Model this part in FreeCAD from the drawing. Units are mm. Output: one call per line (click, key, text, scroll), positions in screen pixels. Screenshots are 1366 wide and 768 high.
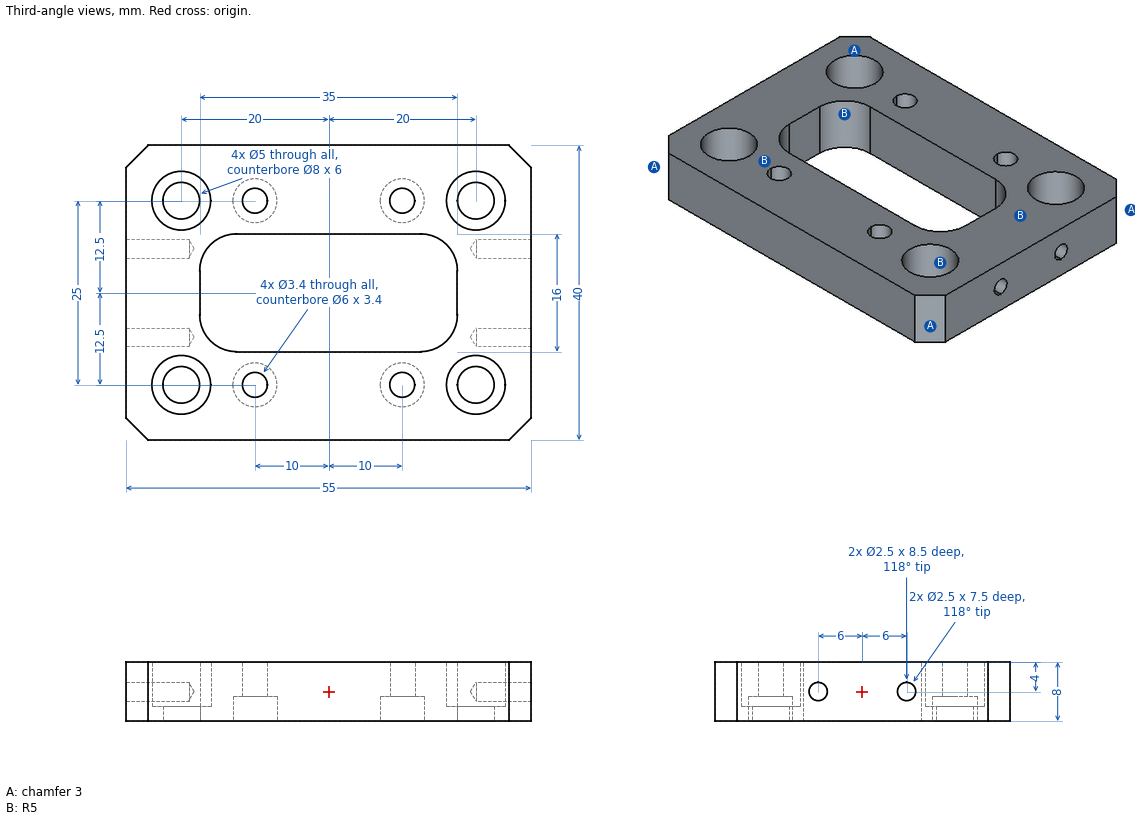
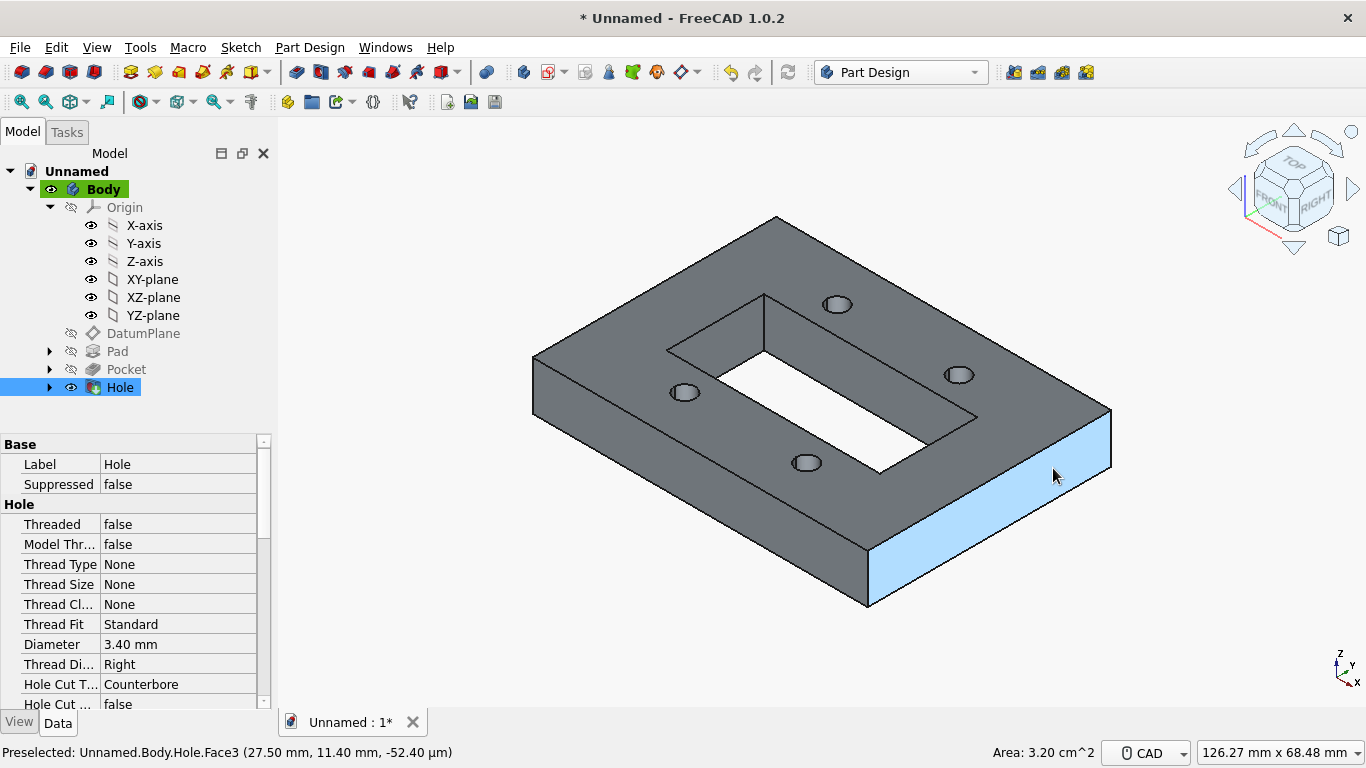
click(548, 72)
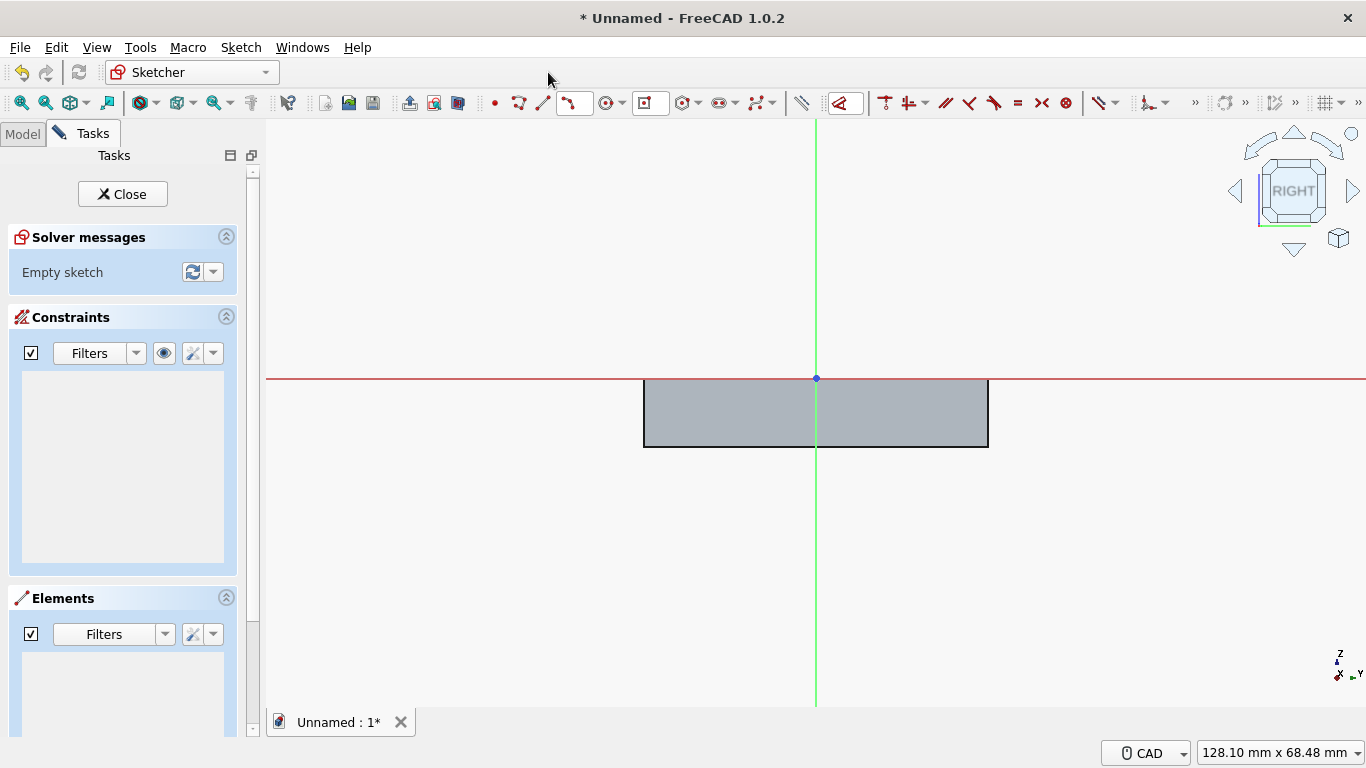
scroll(833, 398, up, 8)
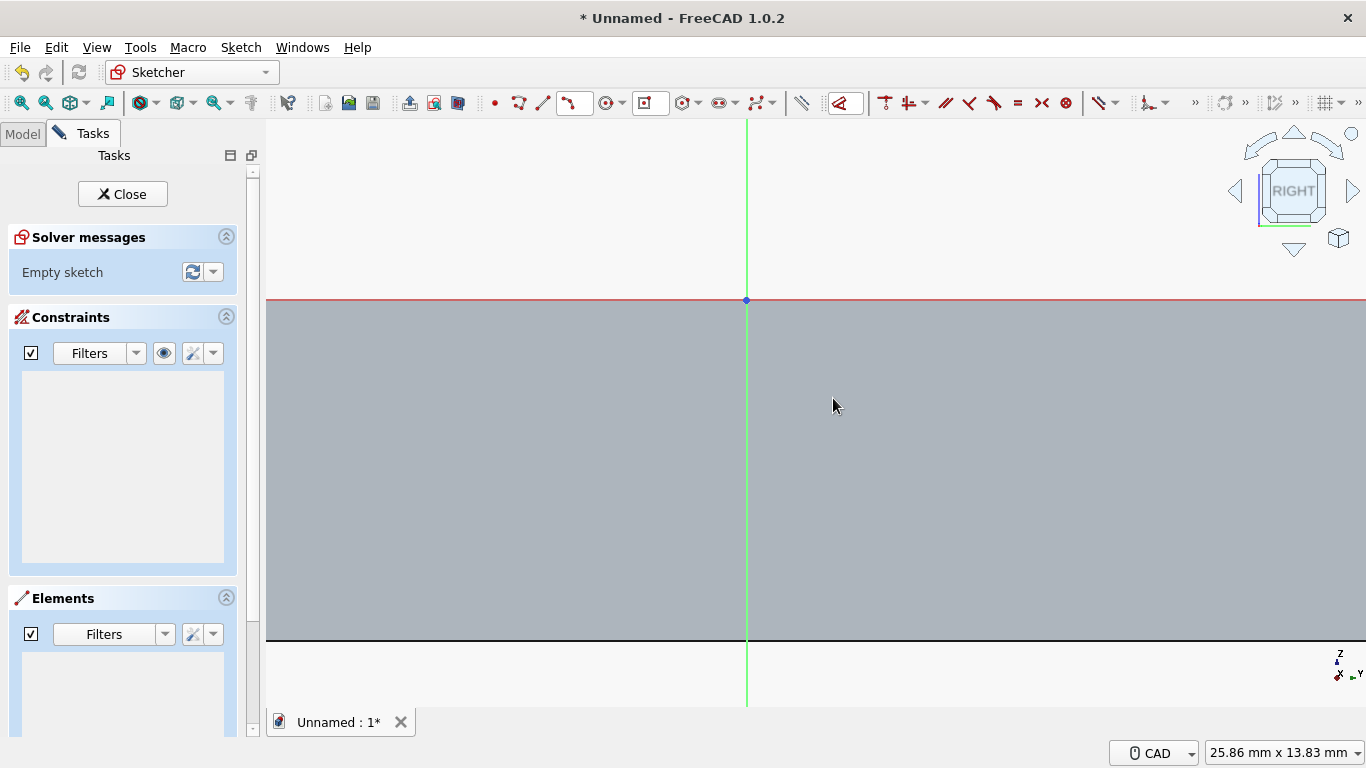
click(606, 104)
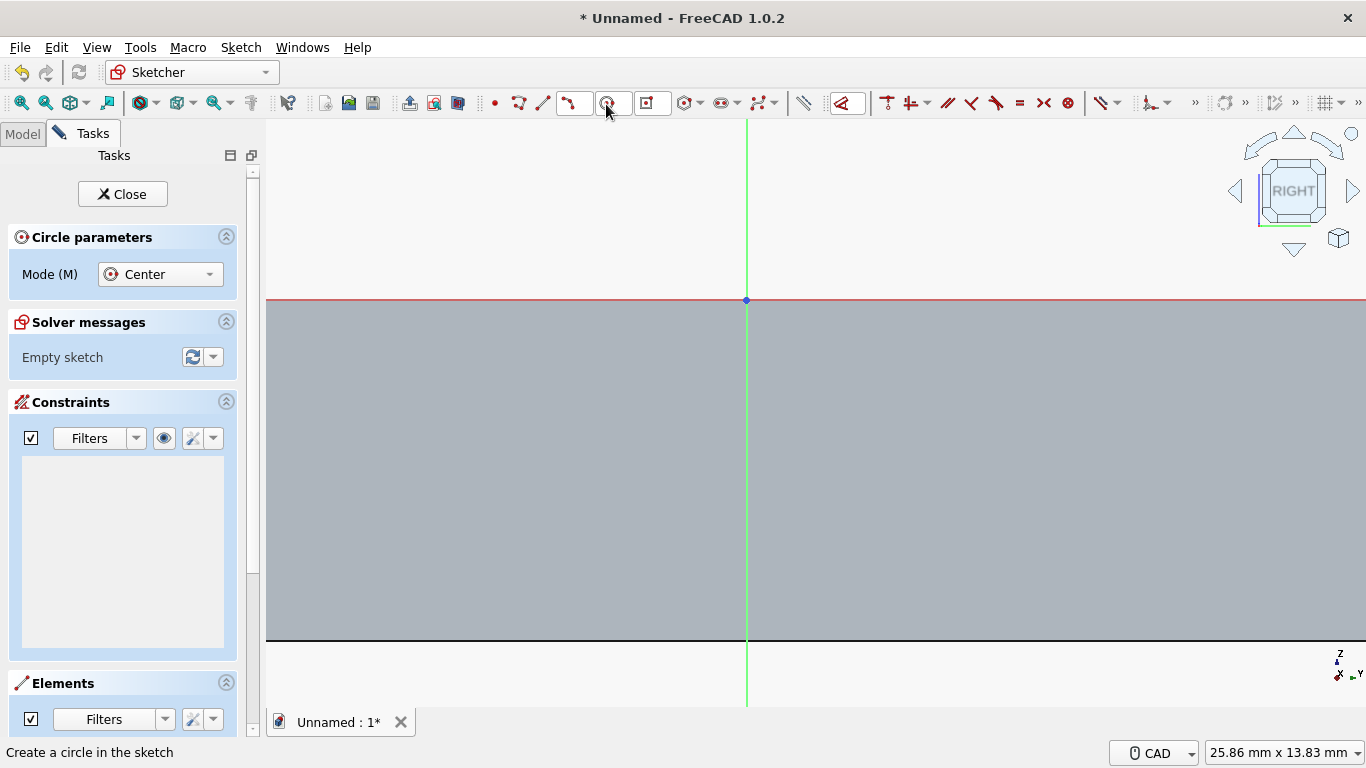
click(1002, 470)
move(1040, 433)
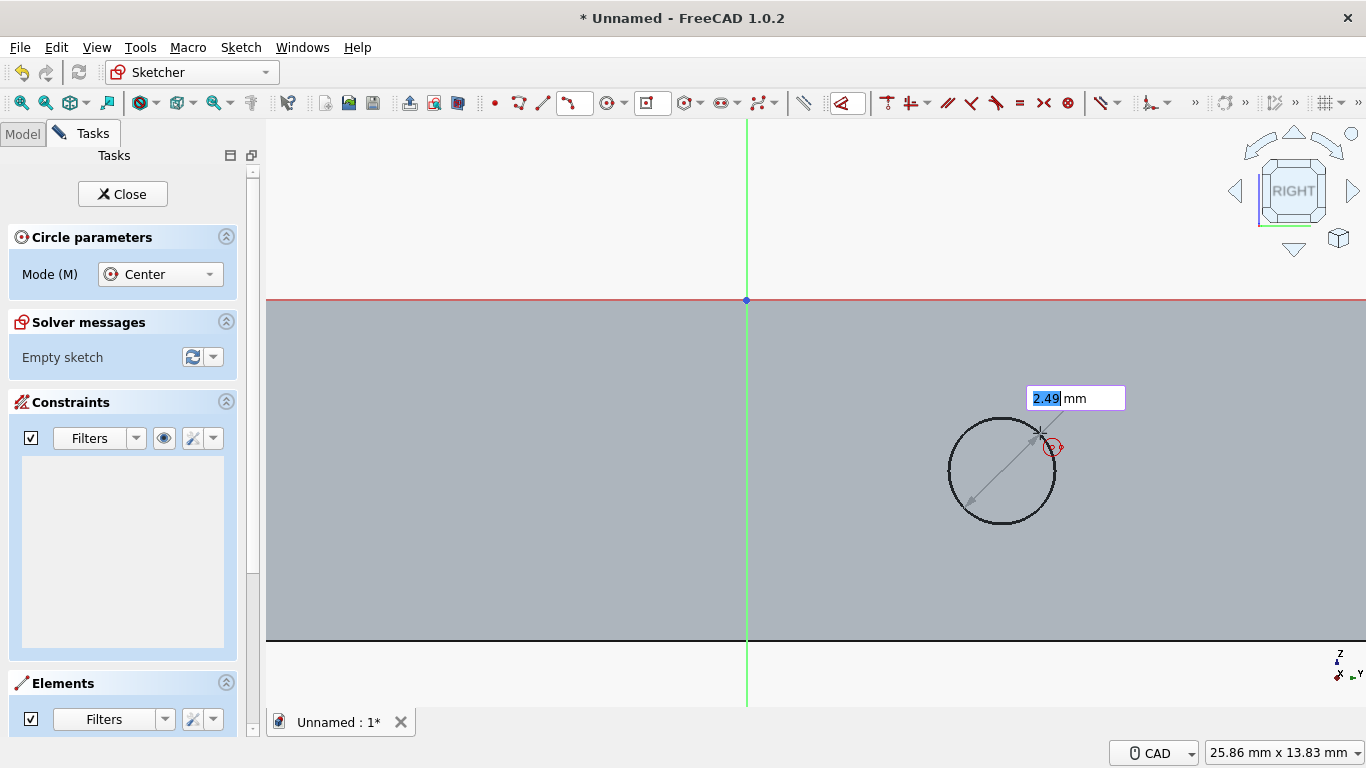
text(2.5)
key(Return)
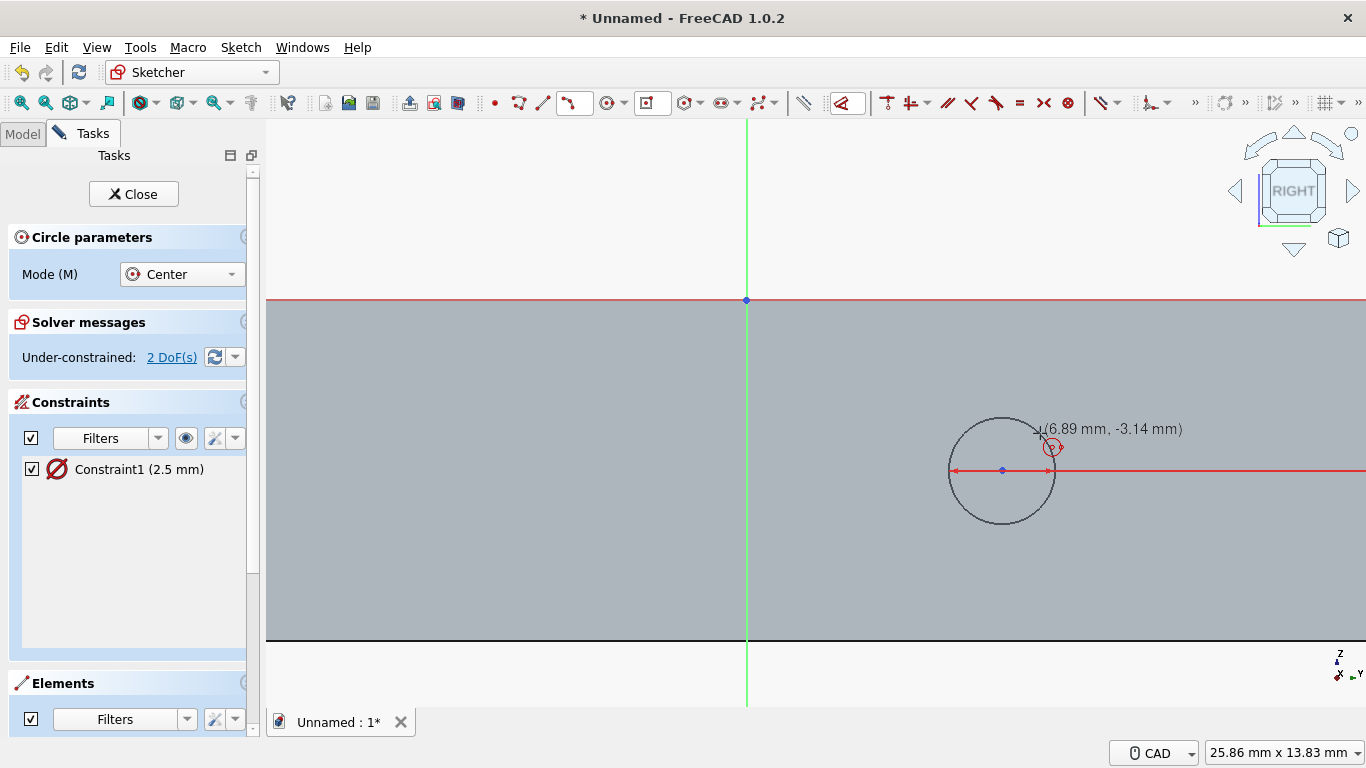
click(492, 470)
move(529, 433)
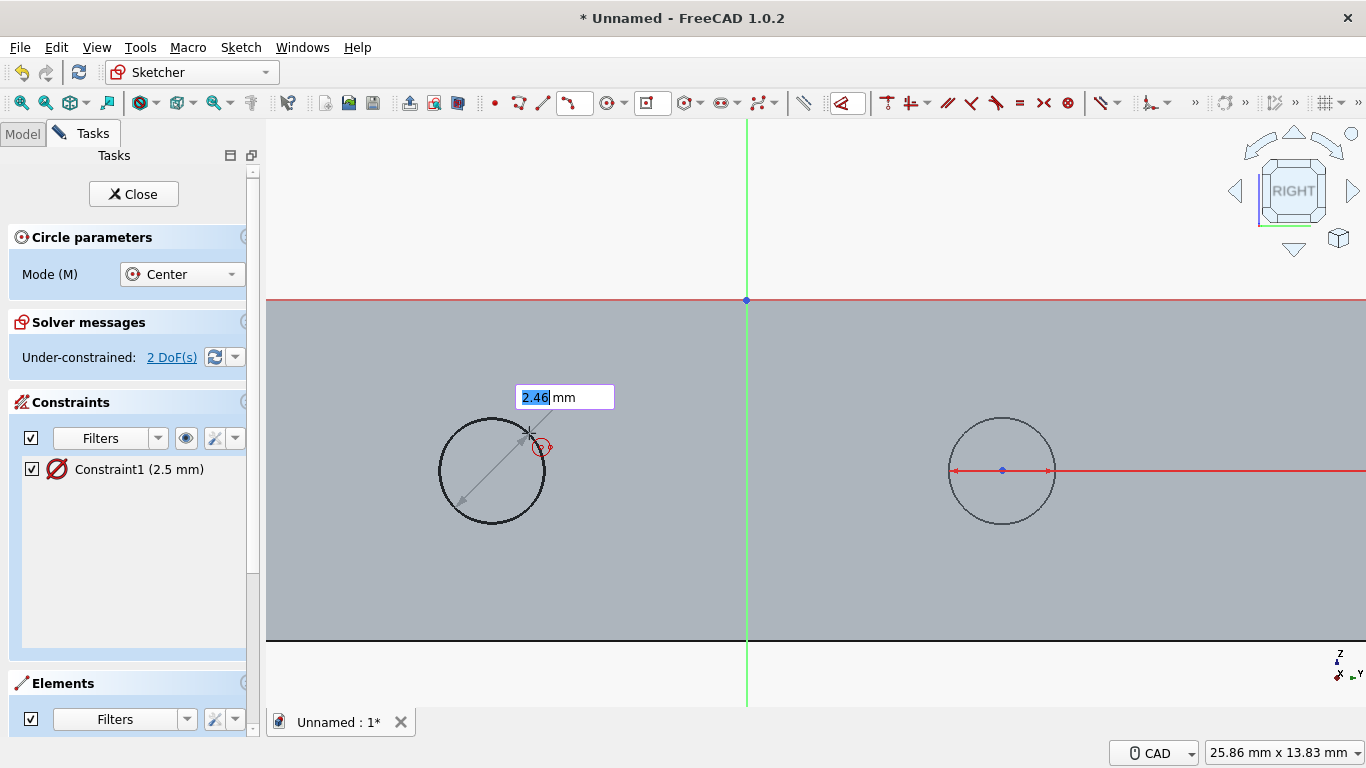
text(2.5)
key(Return)
key(Escape)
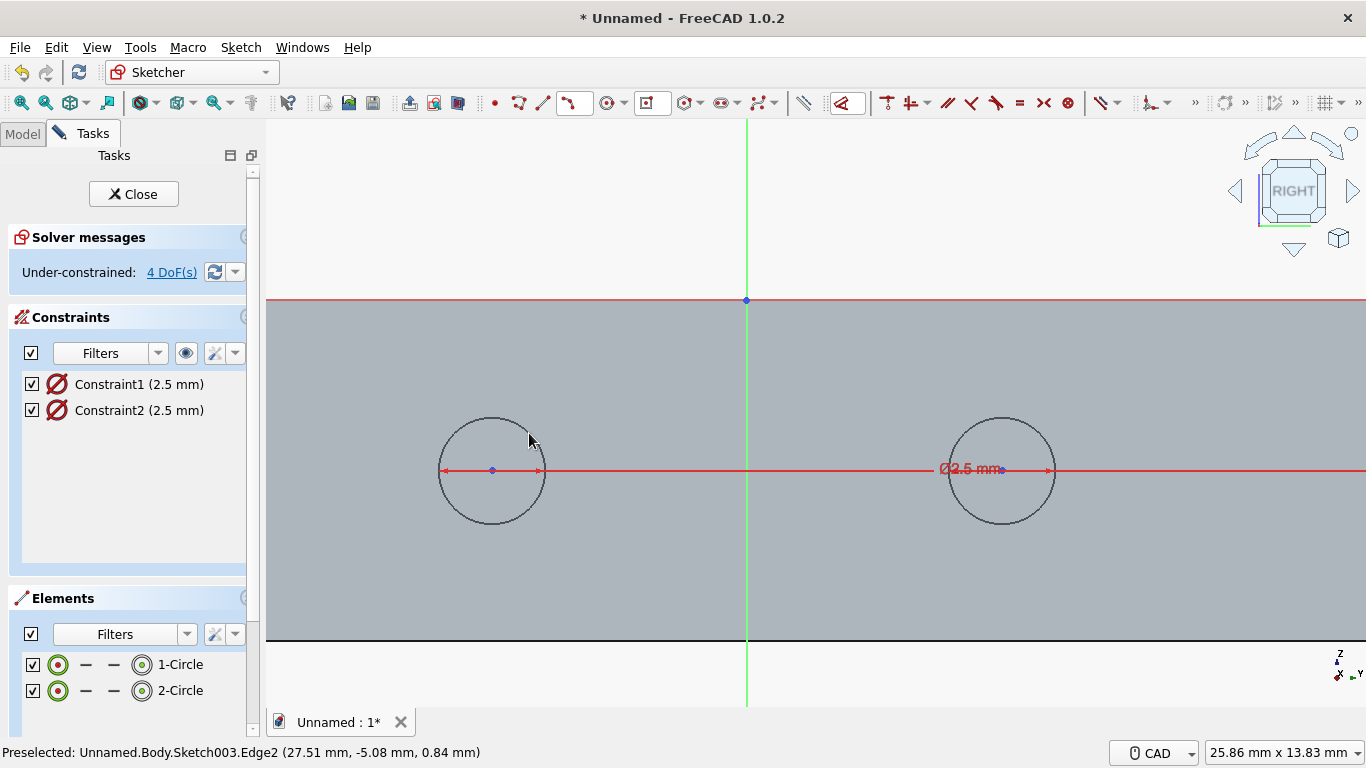
click(1002, 471)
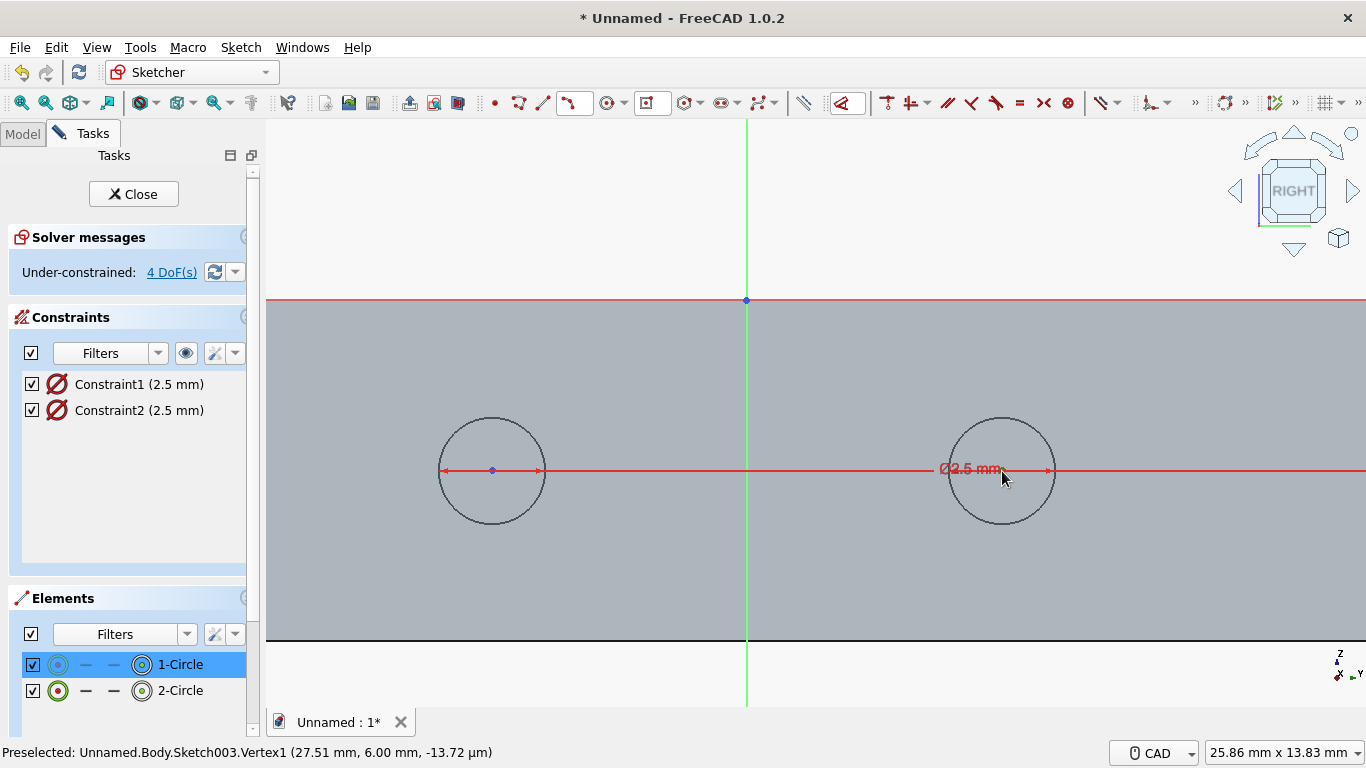
click(492, 471)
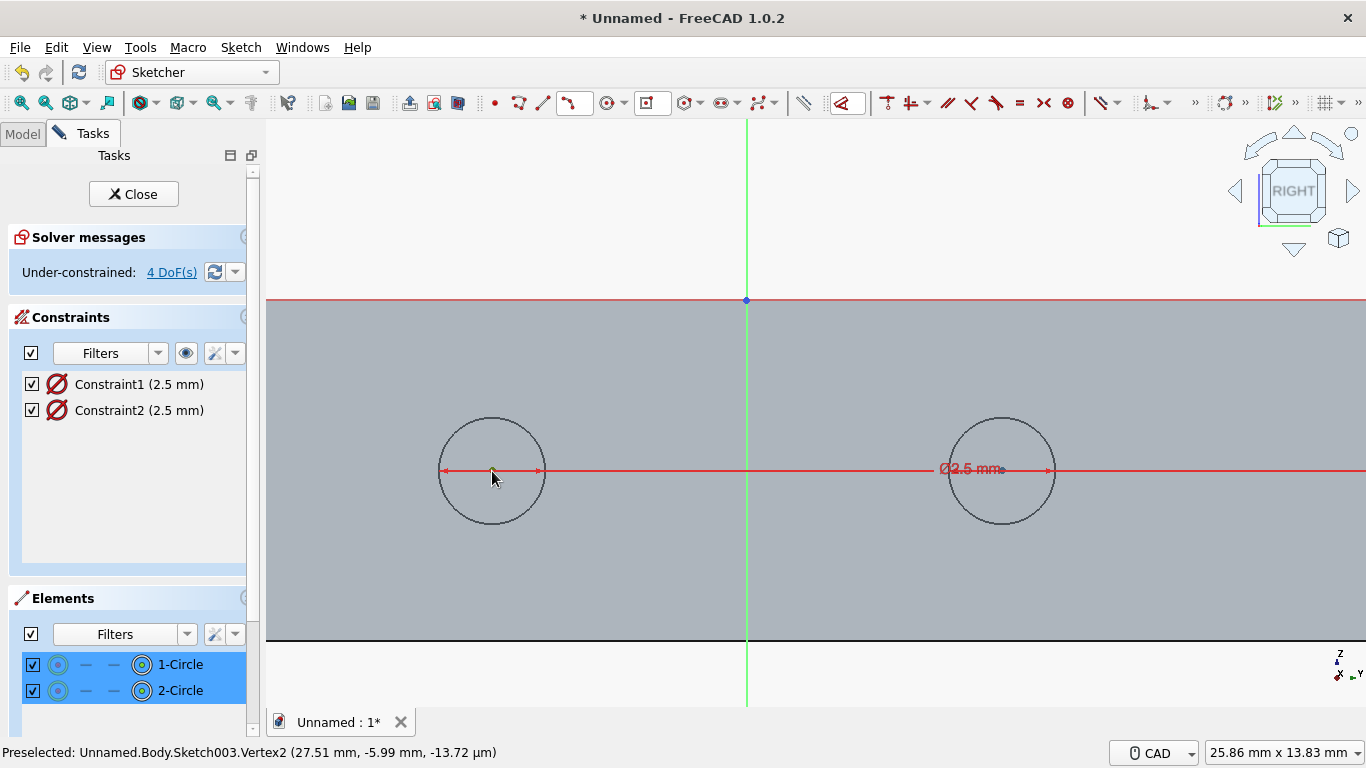
click(930, 104)